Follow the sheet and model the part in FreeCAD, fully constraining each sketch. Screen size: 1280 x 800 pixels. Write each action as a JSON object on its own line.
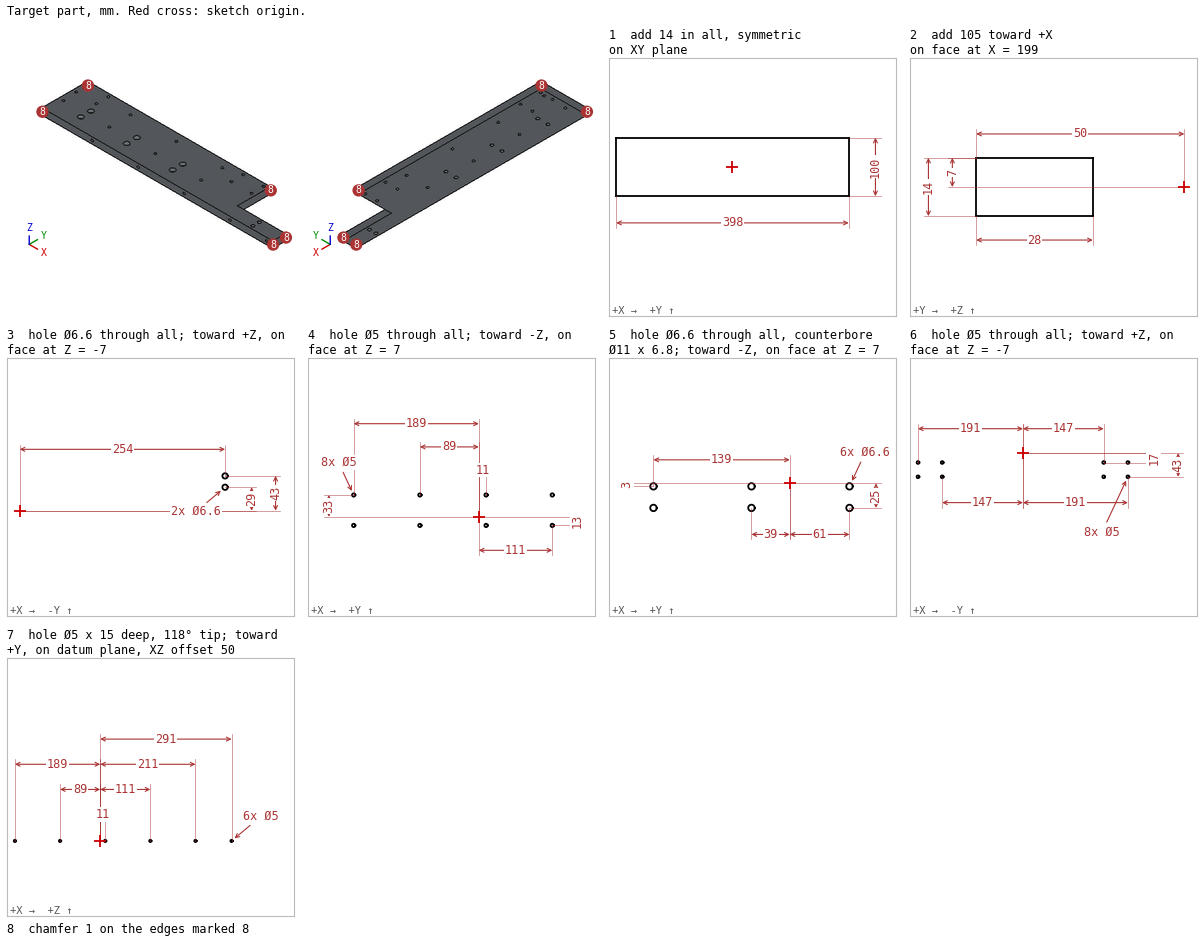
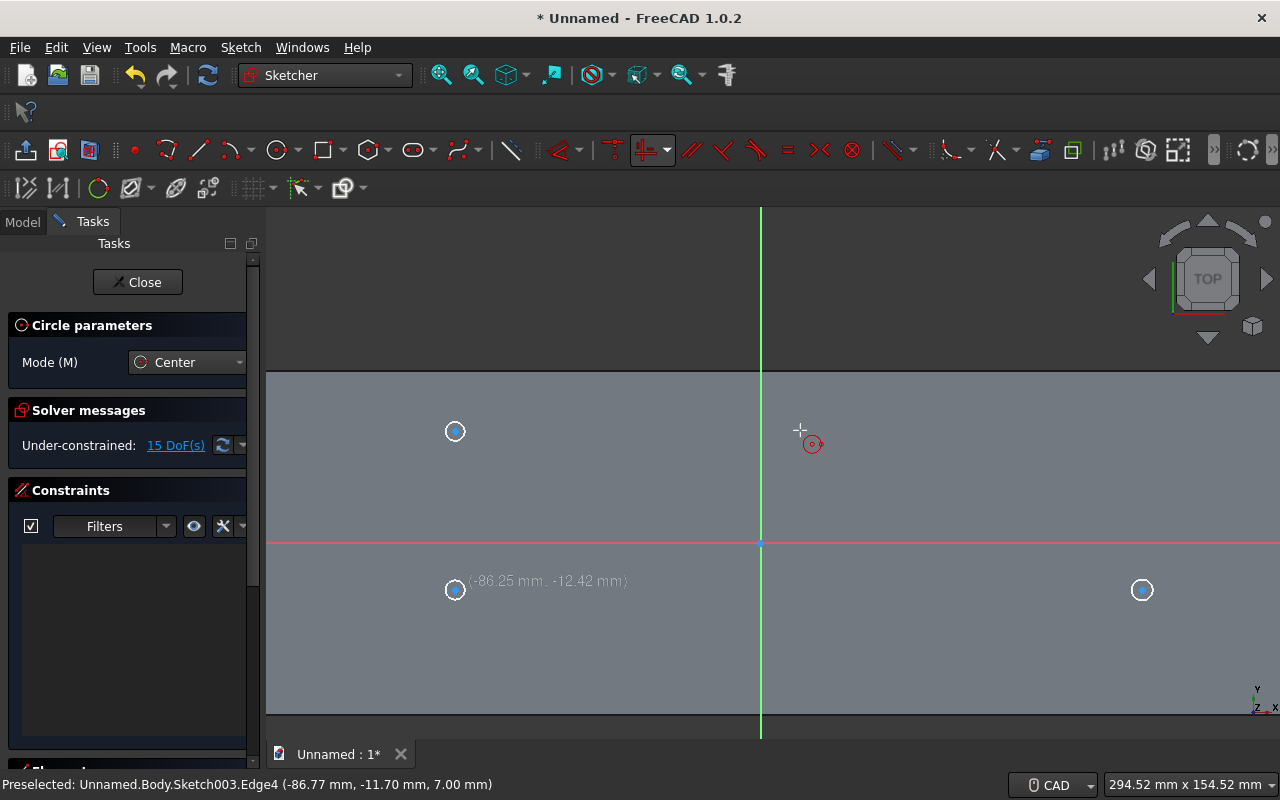
{"action": "left_click", "coordinate": [800, 430]}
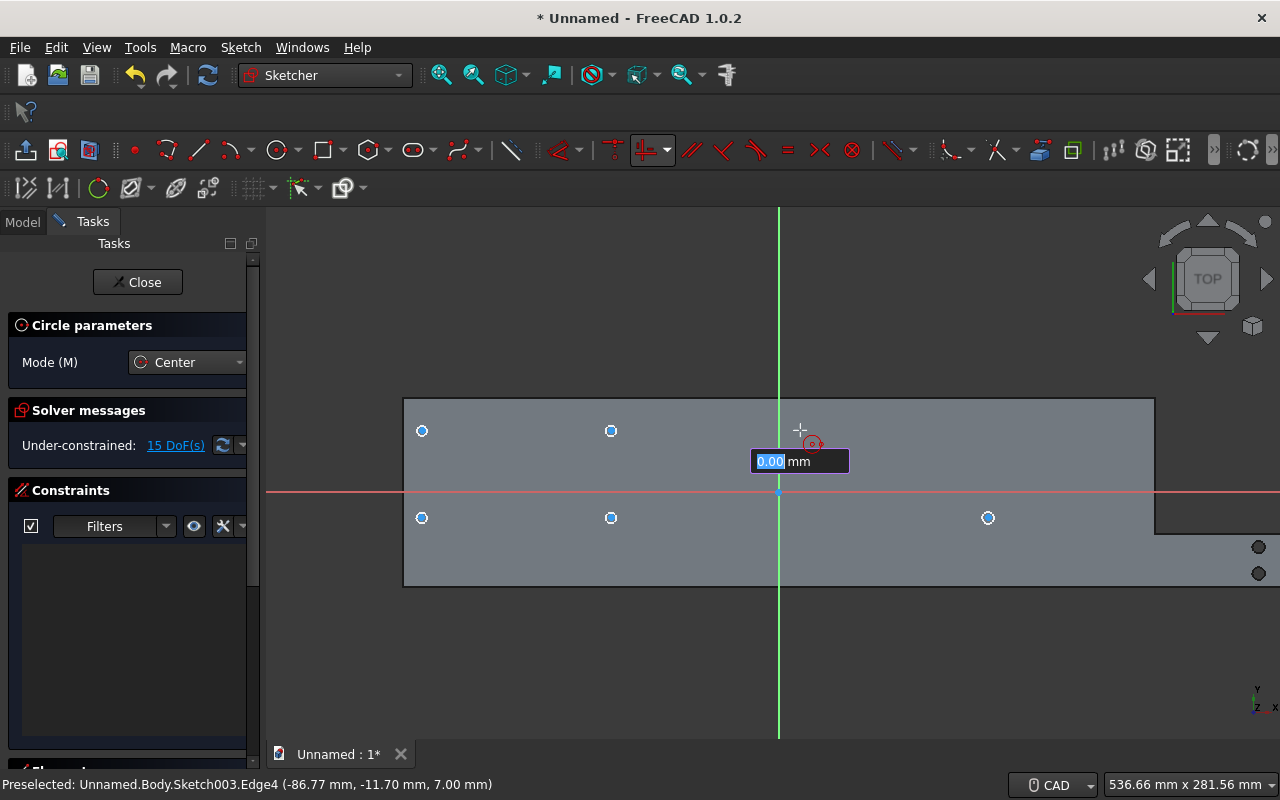
{"action": "scroll", "coordinate": [803, 427], "scroll_direction": "up", "scroll_amount": 7}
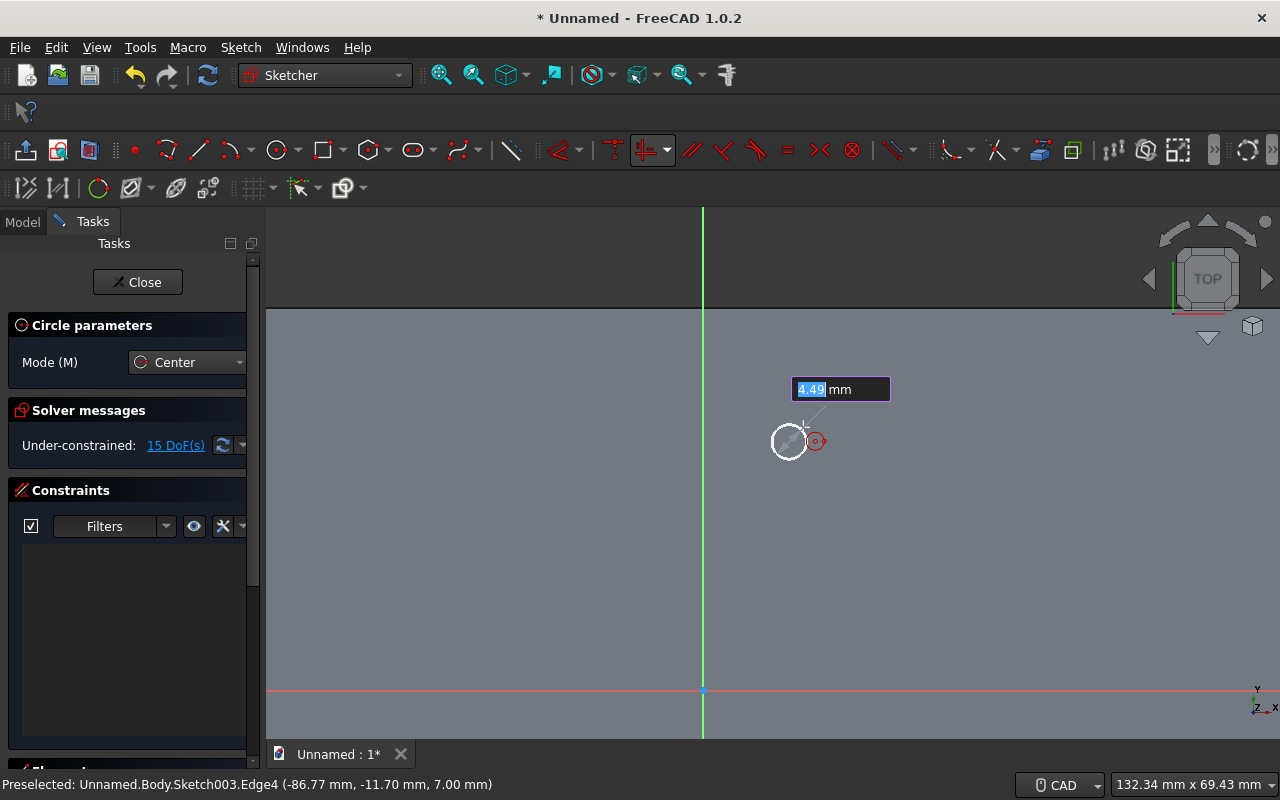
{"action": "left_click", "coordinate": [801, 424]}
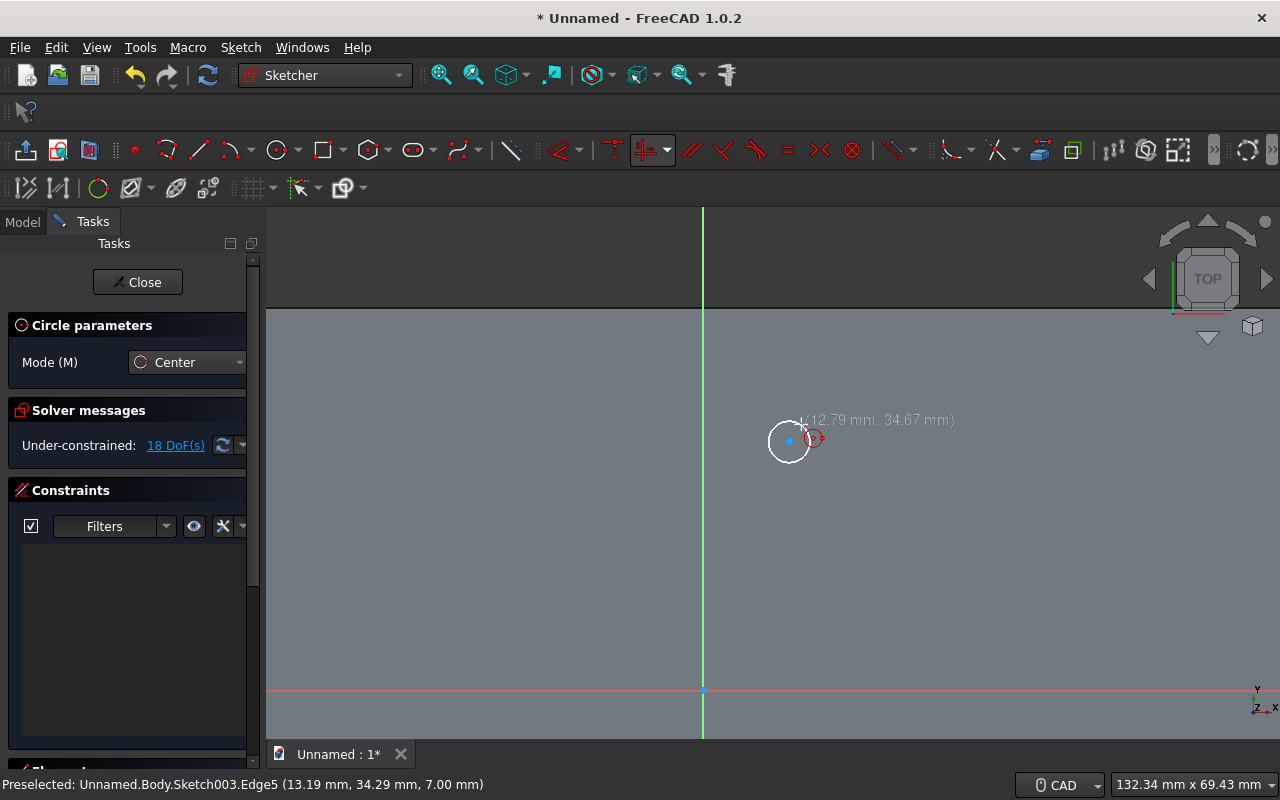
{"action": "scroll", "coordinate": [803, 427], "scroll_direction": "down", "scroll_amount": 7}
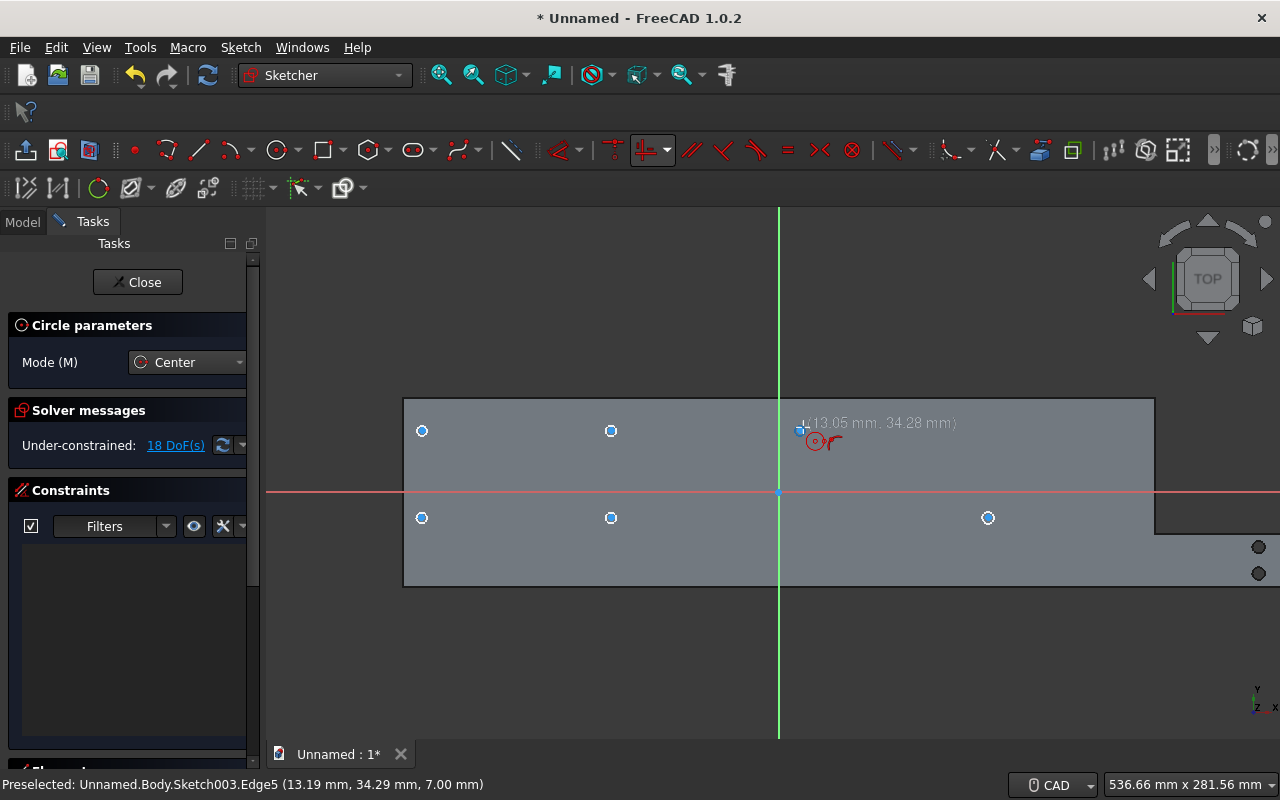
{"action": "scroll", "coordinate": [800, 517], "scroll_direction": "up", "scroll_amount": 8}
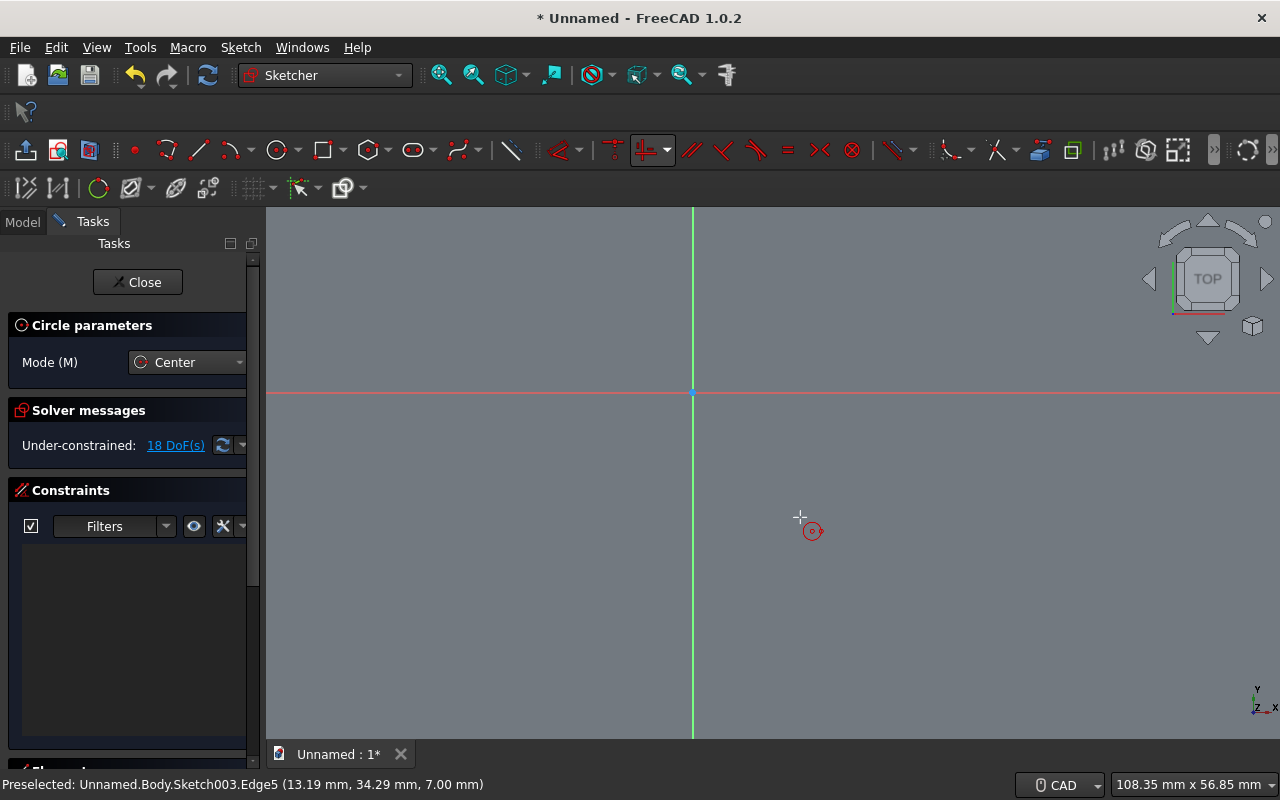
{"action": "scroll", "coordinate": [800, 517], "scroll_direction": "down", "scroll_amount": 8}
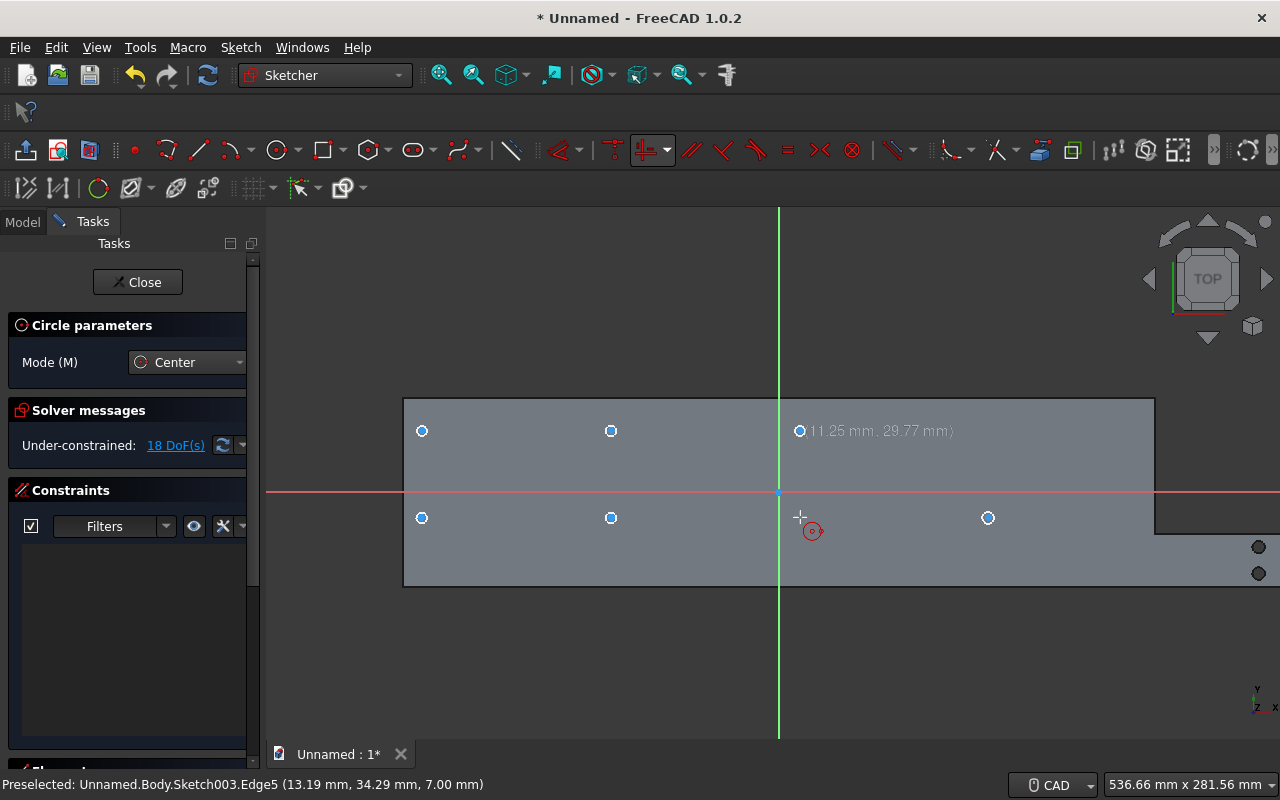
{"action": "left_click", "coordinate": [800, 517]}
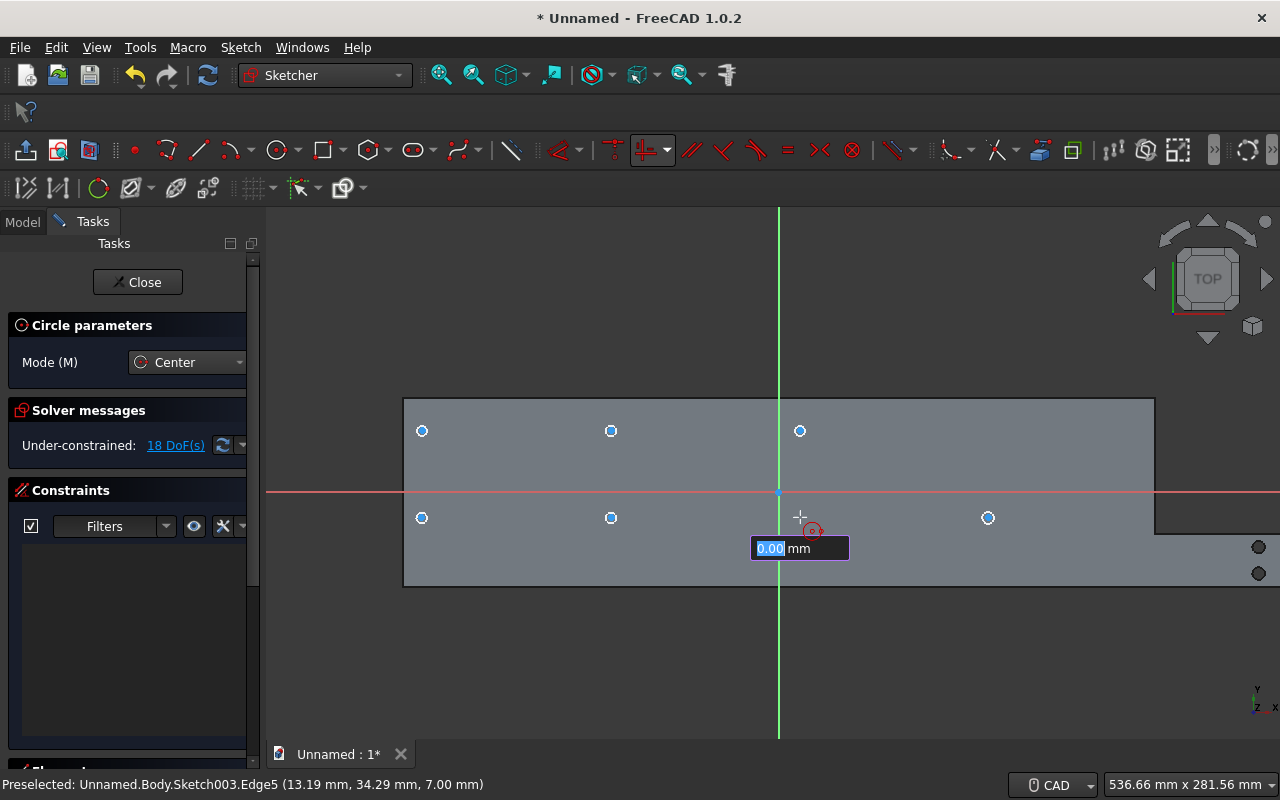
{"action": "scroll", "coordinate": [803, 514], "scroll_direction": "up", "scroll_amount": 7}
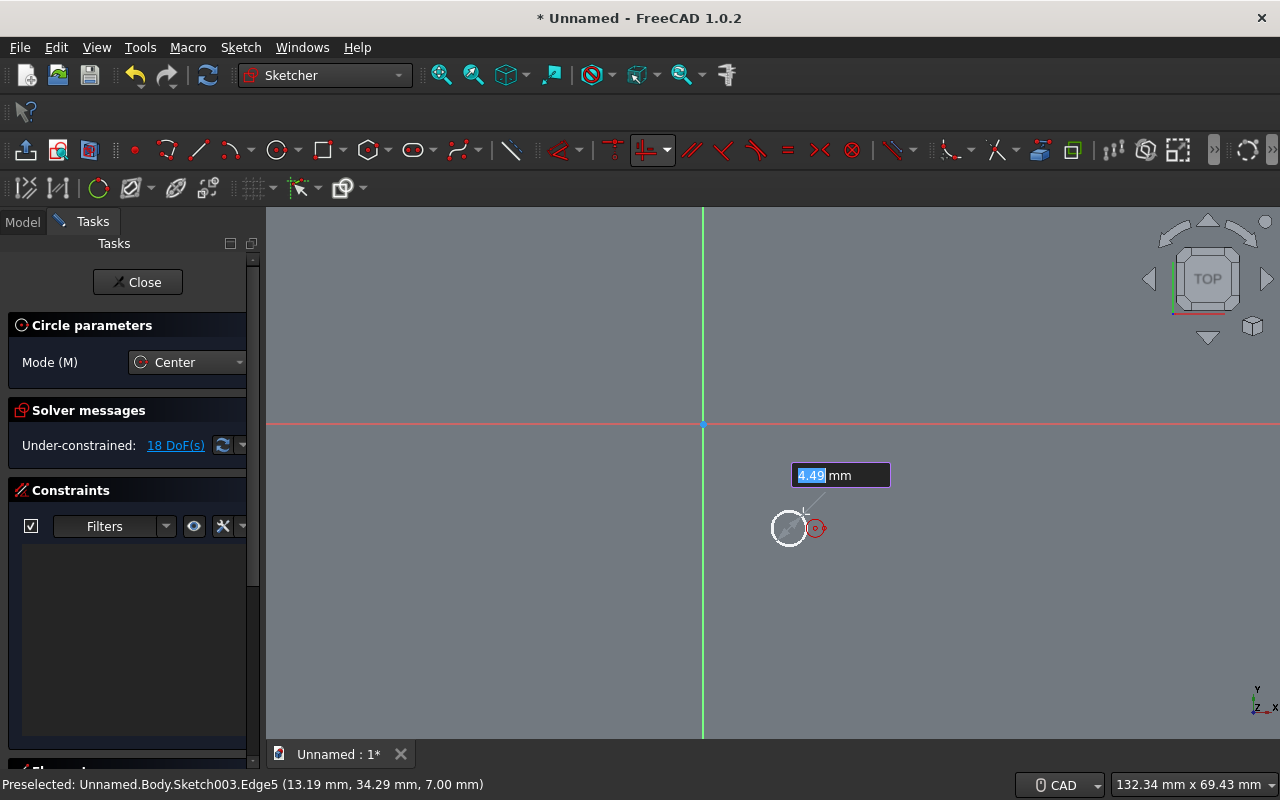
{"action": "left_click", "coordinate": [801, 510]}